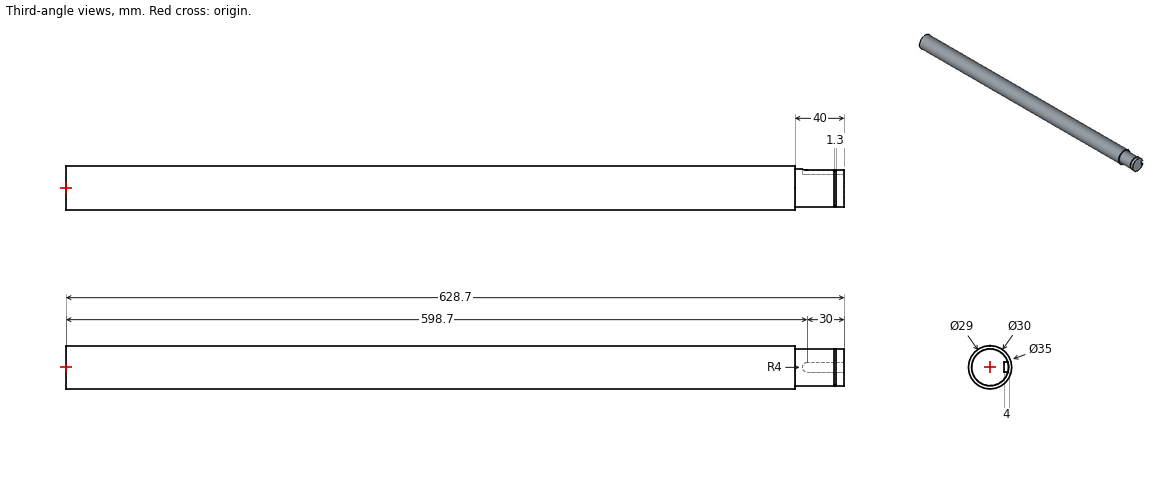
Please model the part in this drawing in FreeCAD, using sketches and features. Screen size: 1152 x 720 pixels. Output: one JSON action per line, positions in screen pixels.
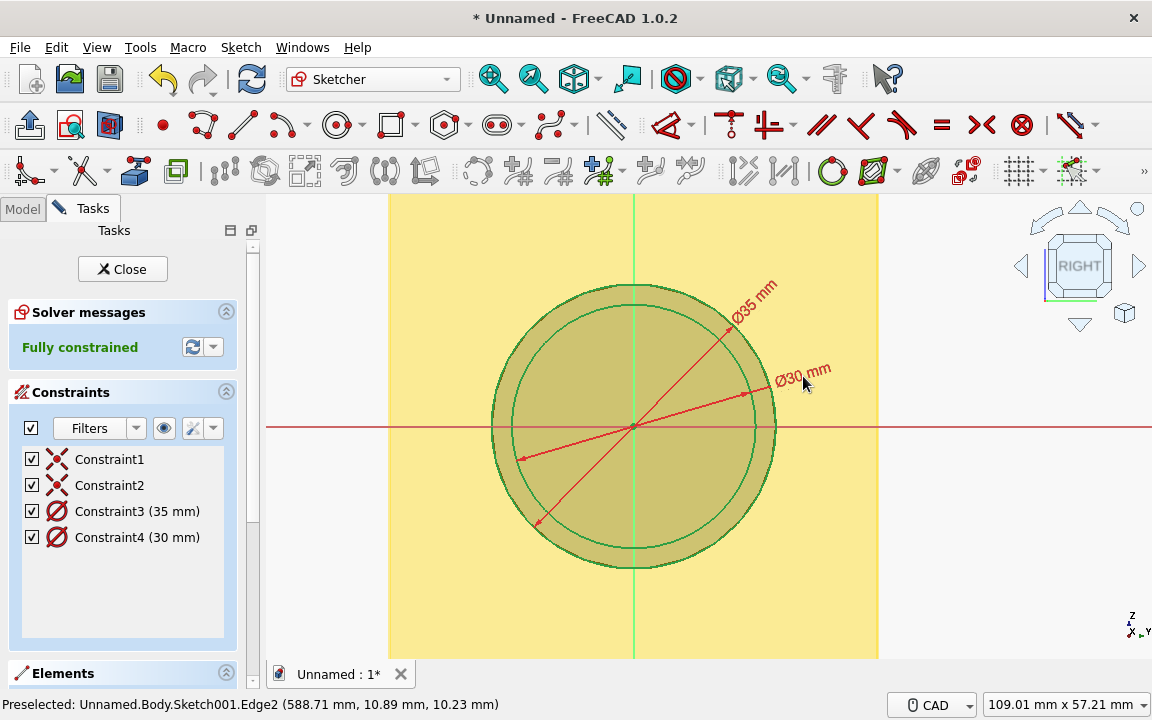
{"action": "left_click", "coordinate": [123, 269]}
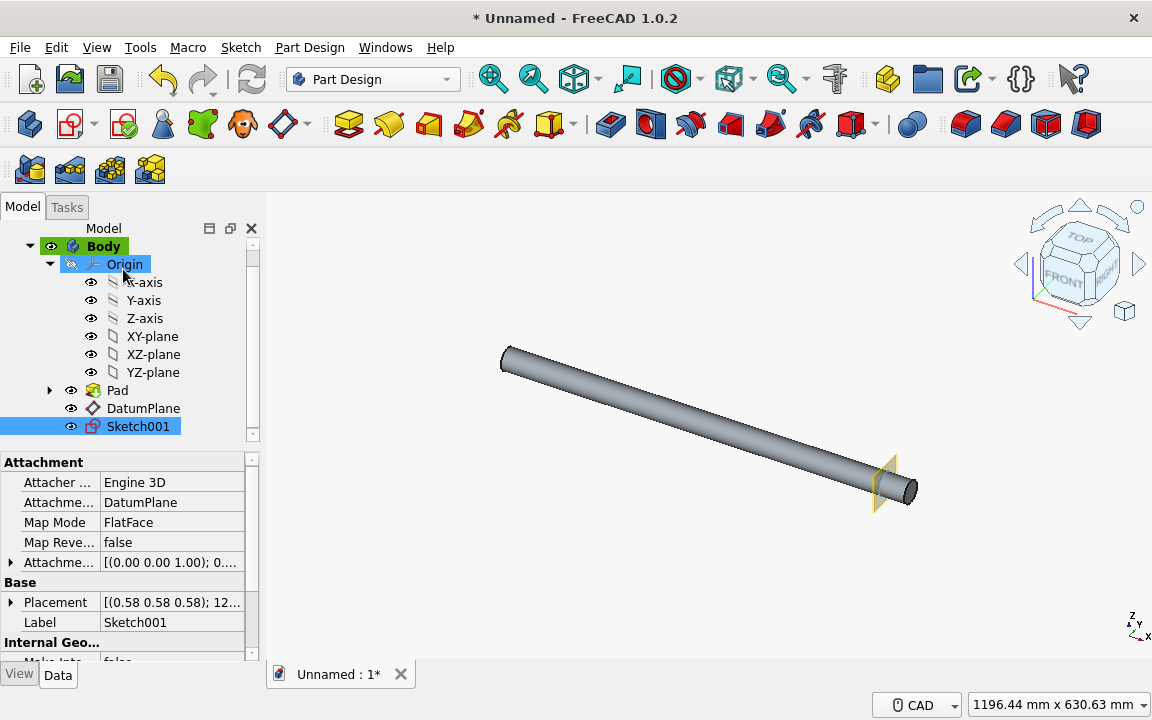
{"action": "left_click", "coordinate": [612, 124]}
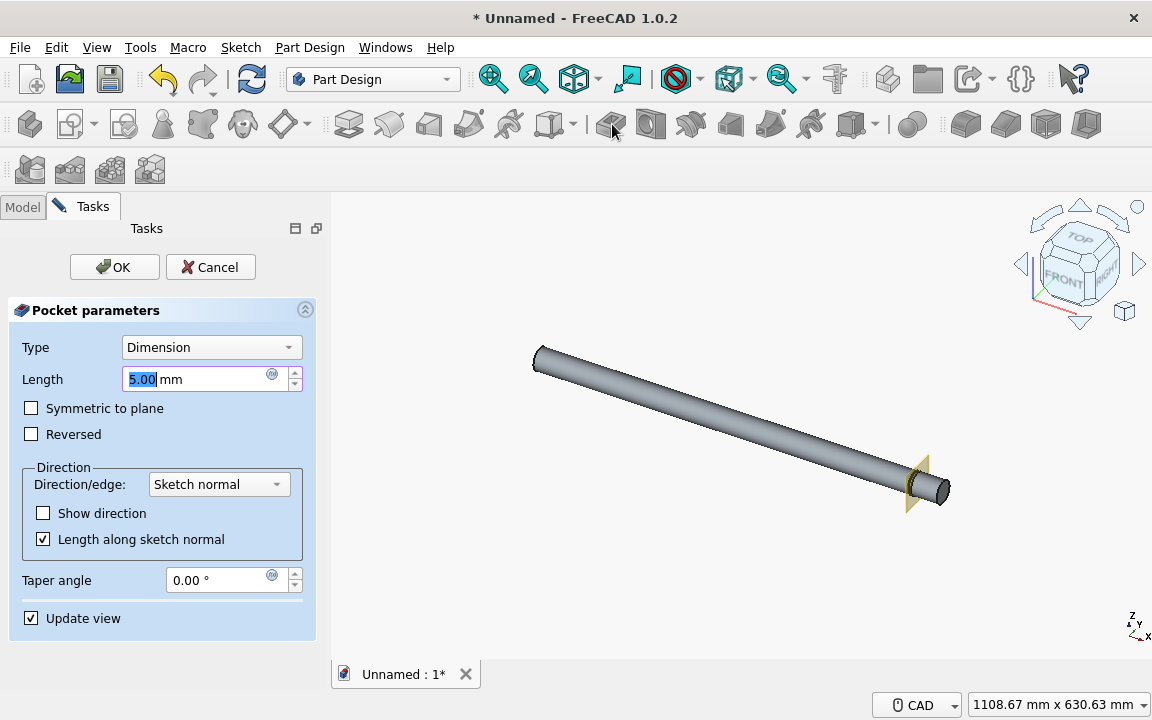
{"action": "type", "text": "40"}
{"action": "key", "text": "Tab"}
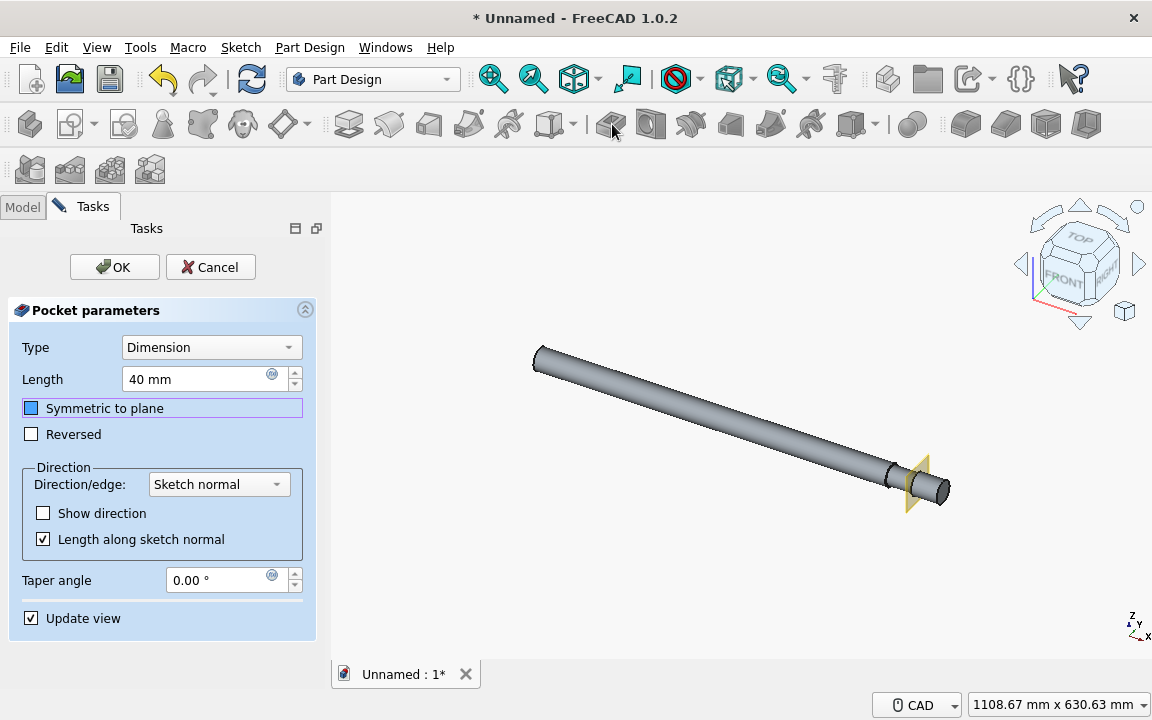
{"action": "left_click", "coordinate": [30, 434]}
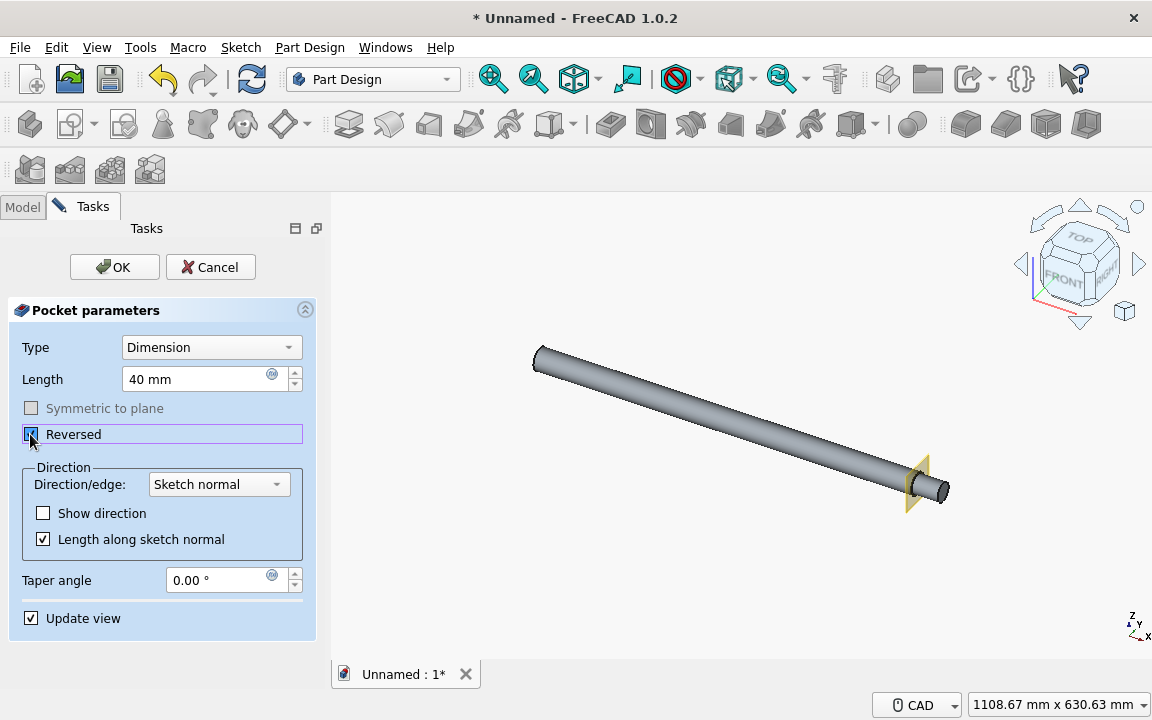
{"action": "left_click", "coordinate": [115, 267]}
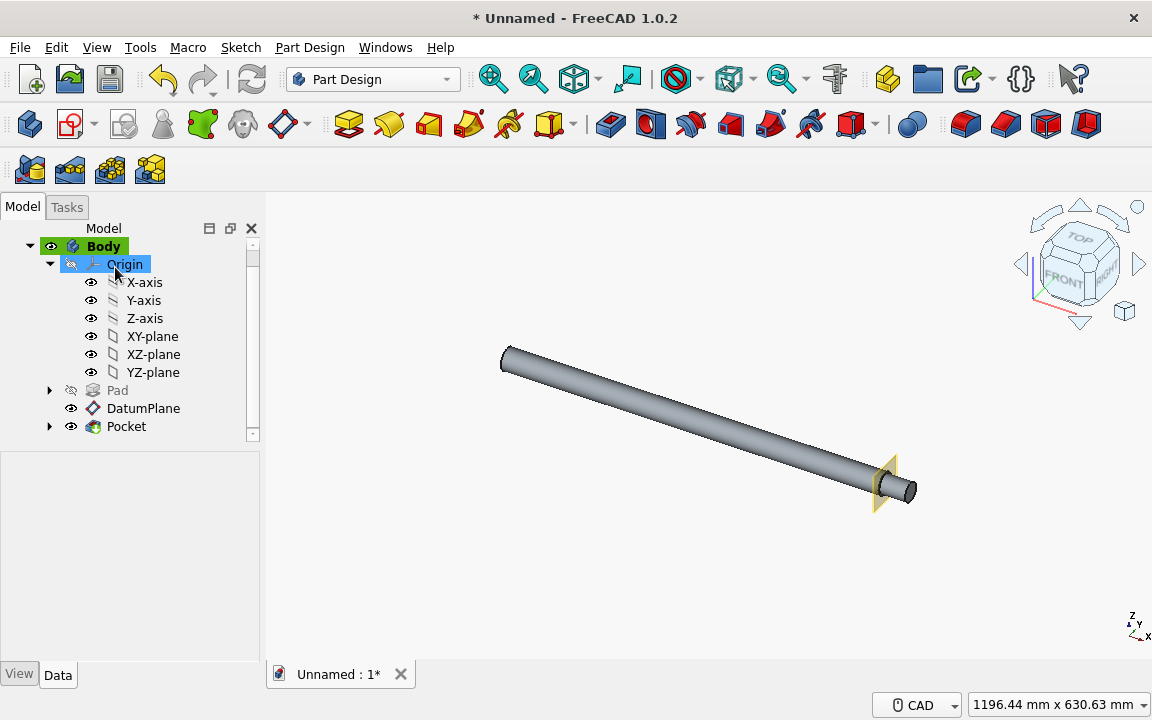
{"action": "left_click", "coordinate": [116, 408]}
{"action": "key", "text": "space"}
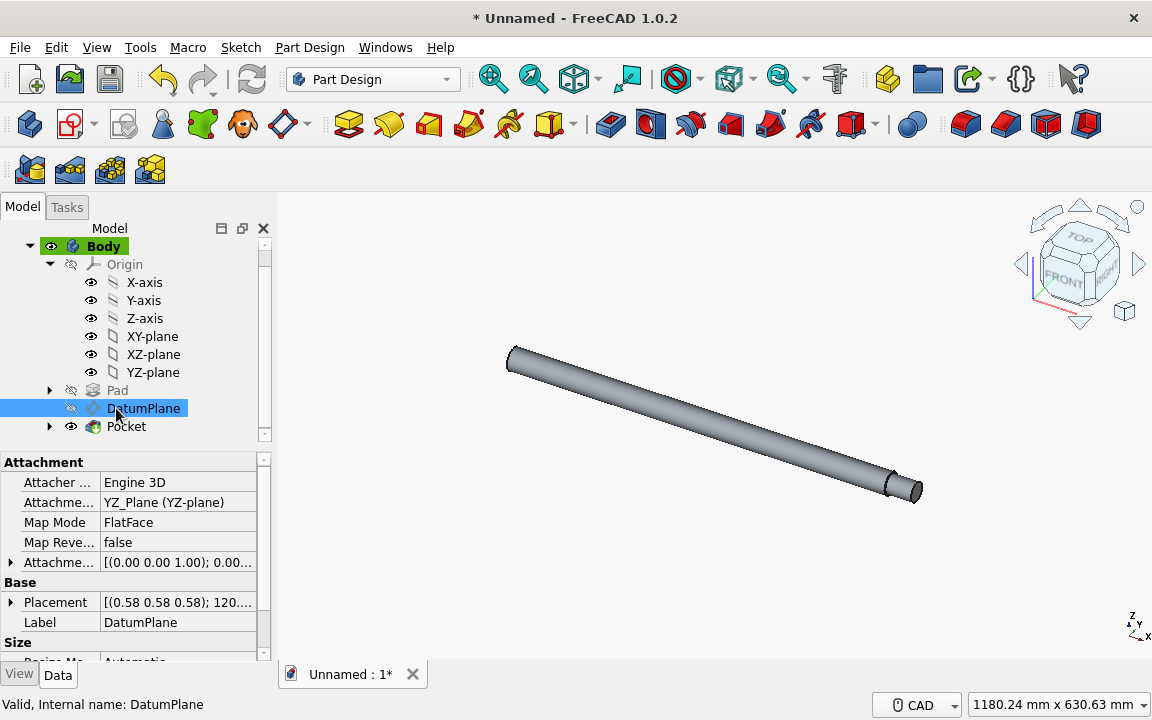
{"action": "left_click", "coordinate": [136, 354]}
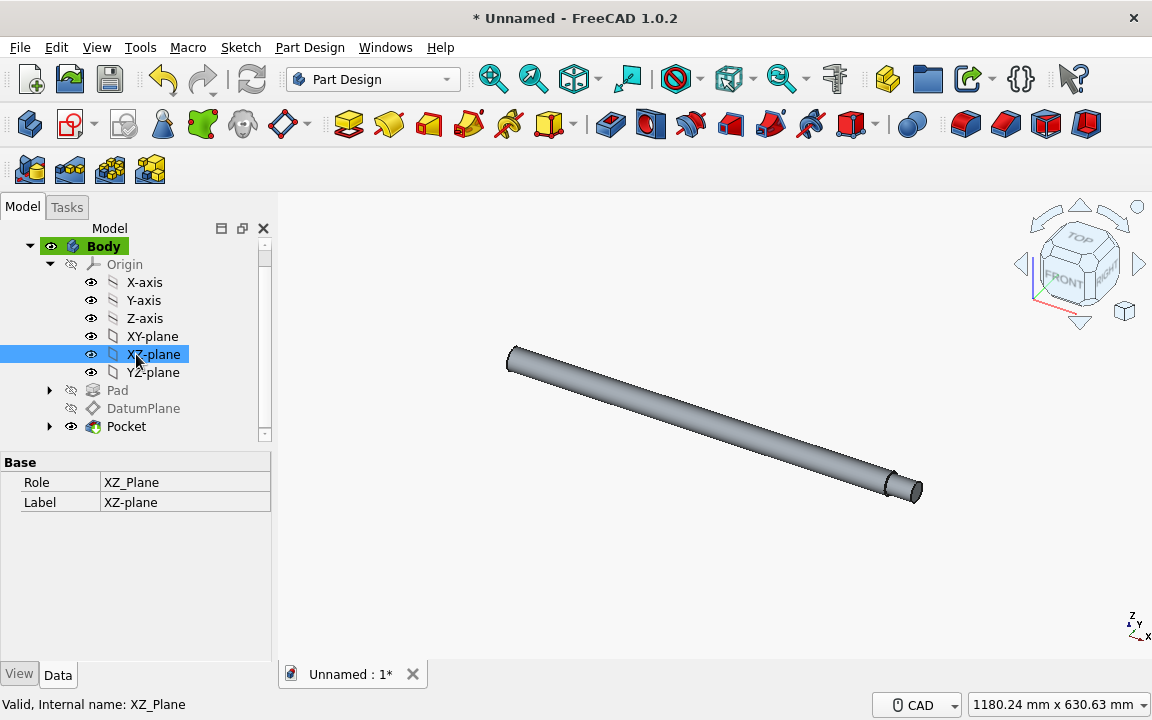
{"action": "left_click", "coordinate": [284, 124]}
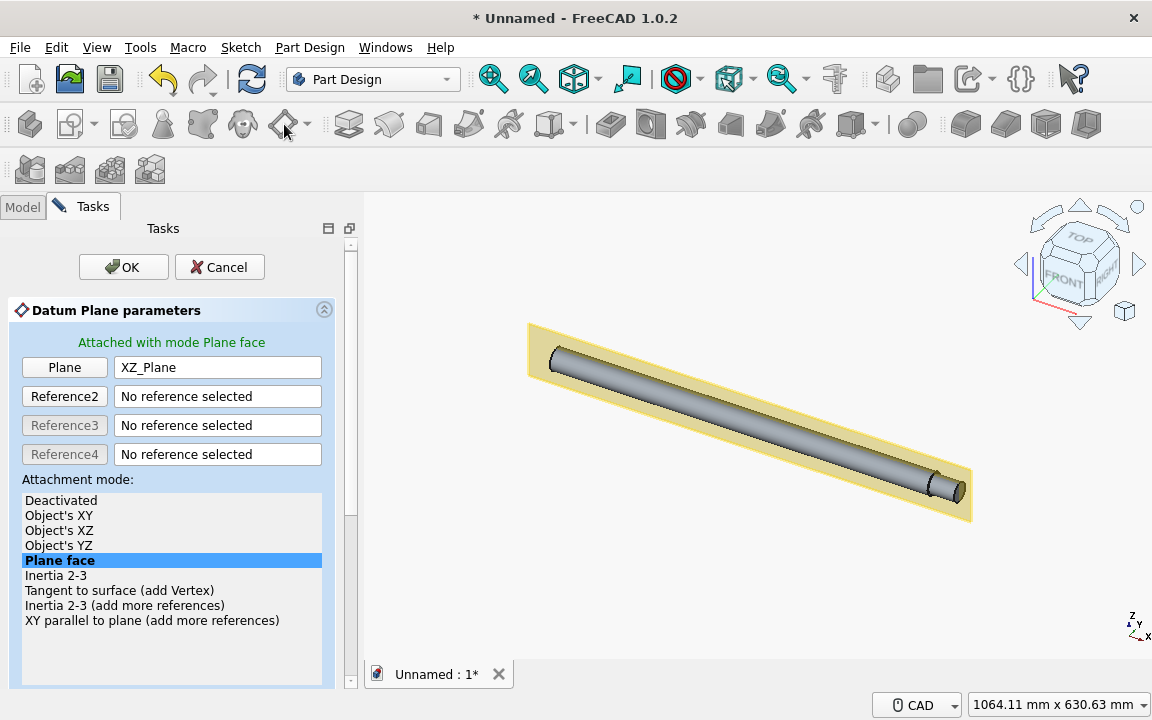
{"action": "scroll", "coordinate": [351, 463], "scroll_direction": "down", "scroll_amount": 3}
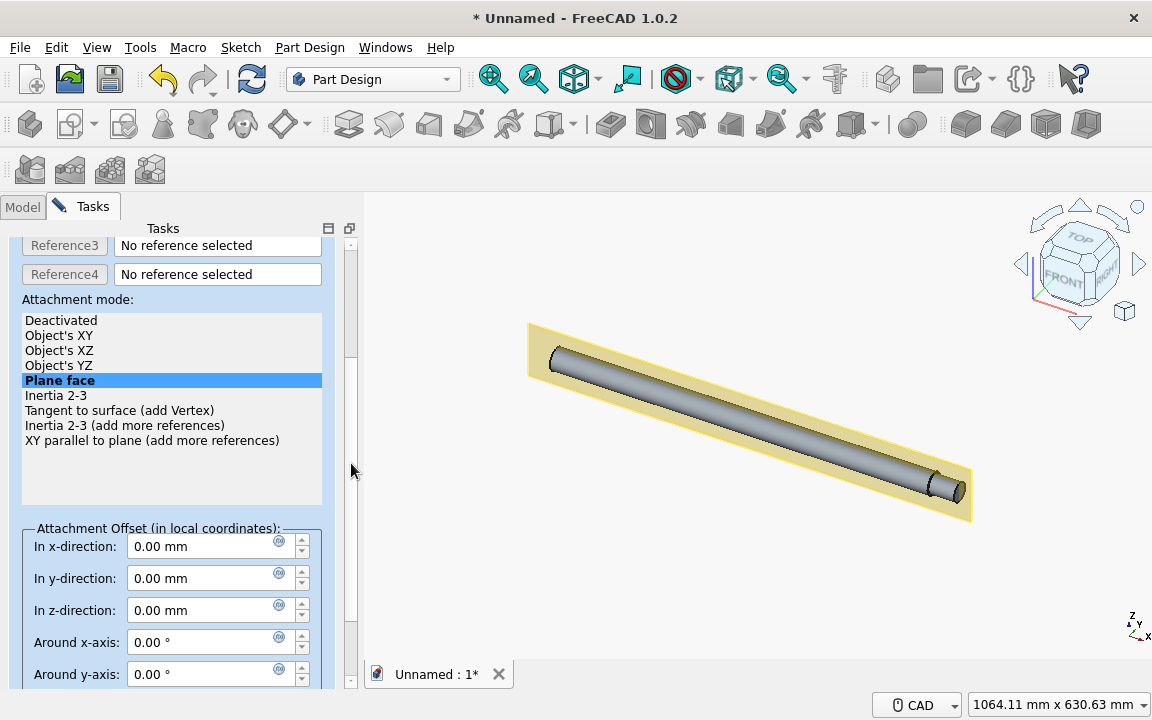
{"action": "triple_click", "coordinate": [210, 610]}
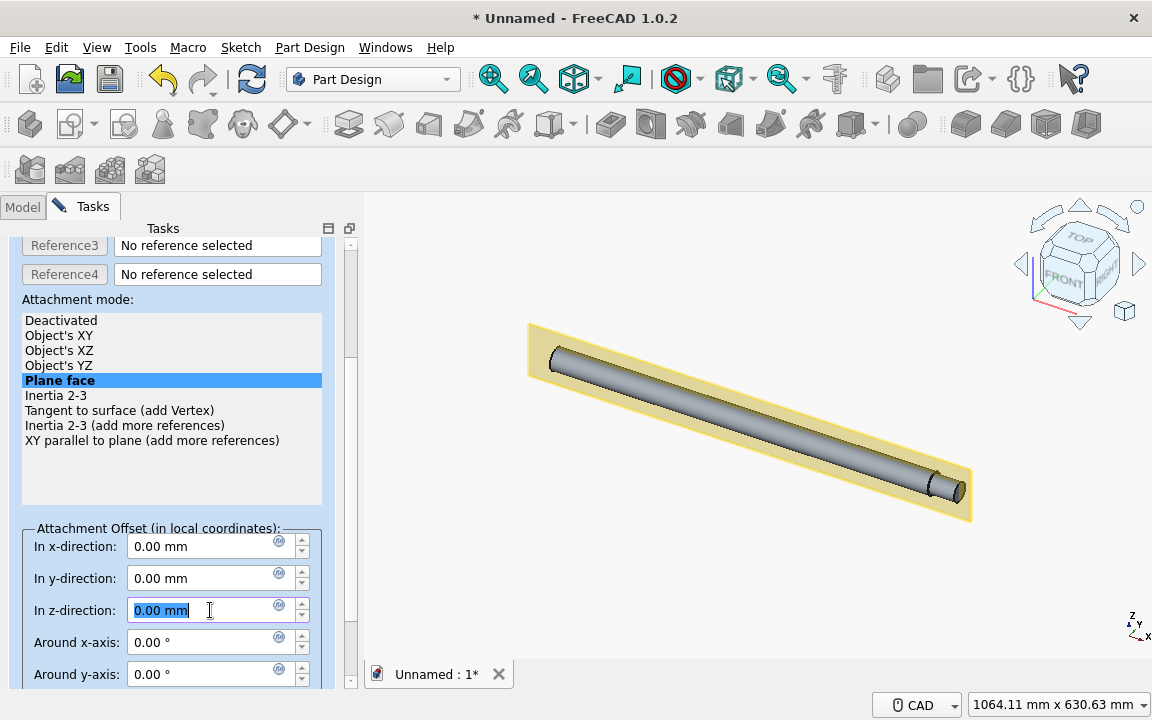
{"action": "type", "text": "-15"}
{"action": "key", "text": "Tab"}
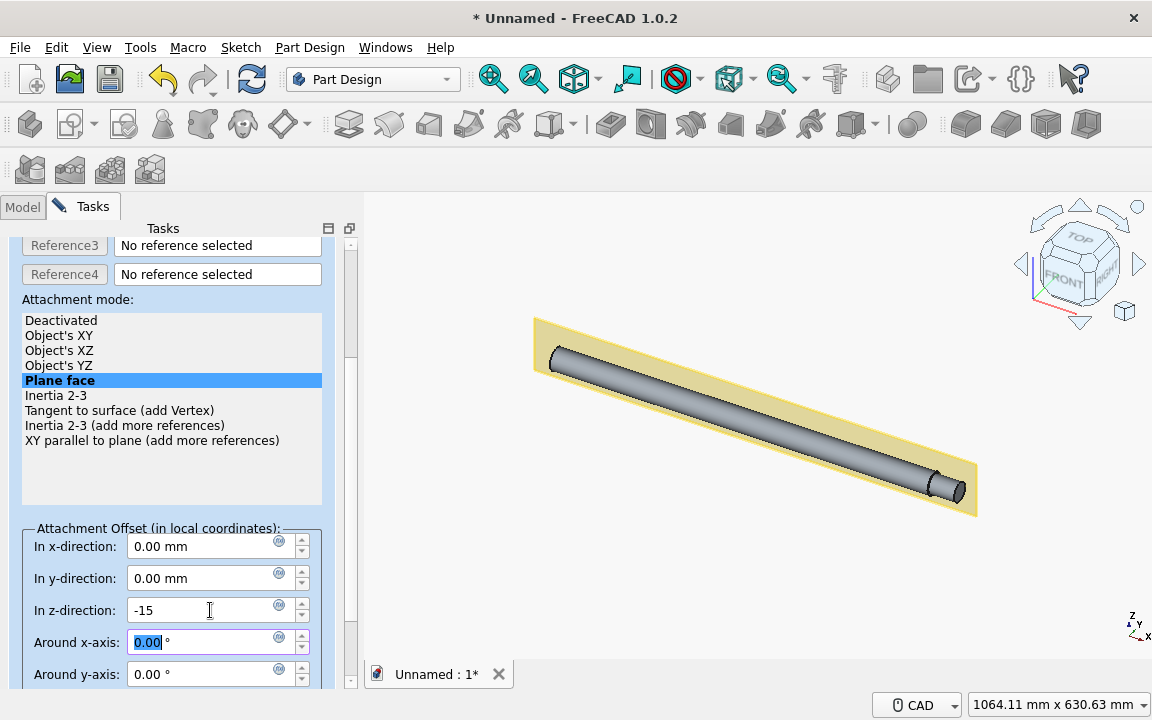
{"action": "scroll", "coordinate": [351, 463], "scroll_direction": "up", "scroll_amount": 4}